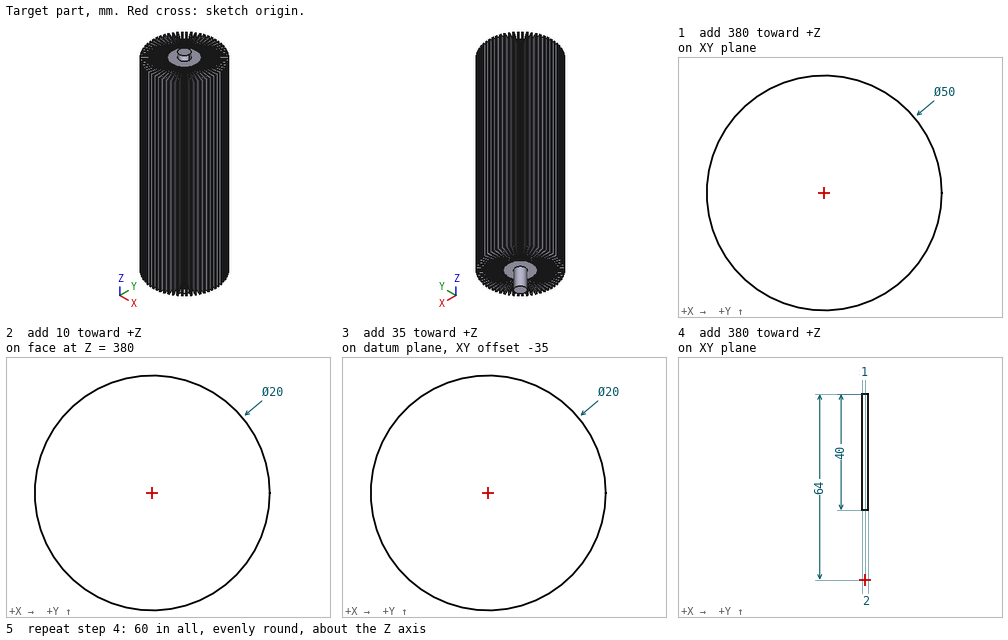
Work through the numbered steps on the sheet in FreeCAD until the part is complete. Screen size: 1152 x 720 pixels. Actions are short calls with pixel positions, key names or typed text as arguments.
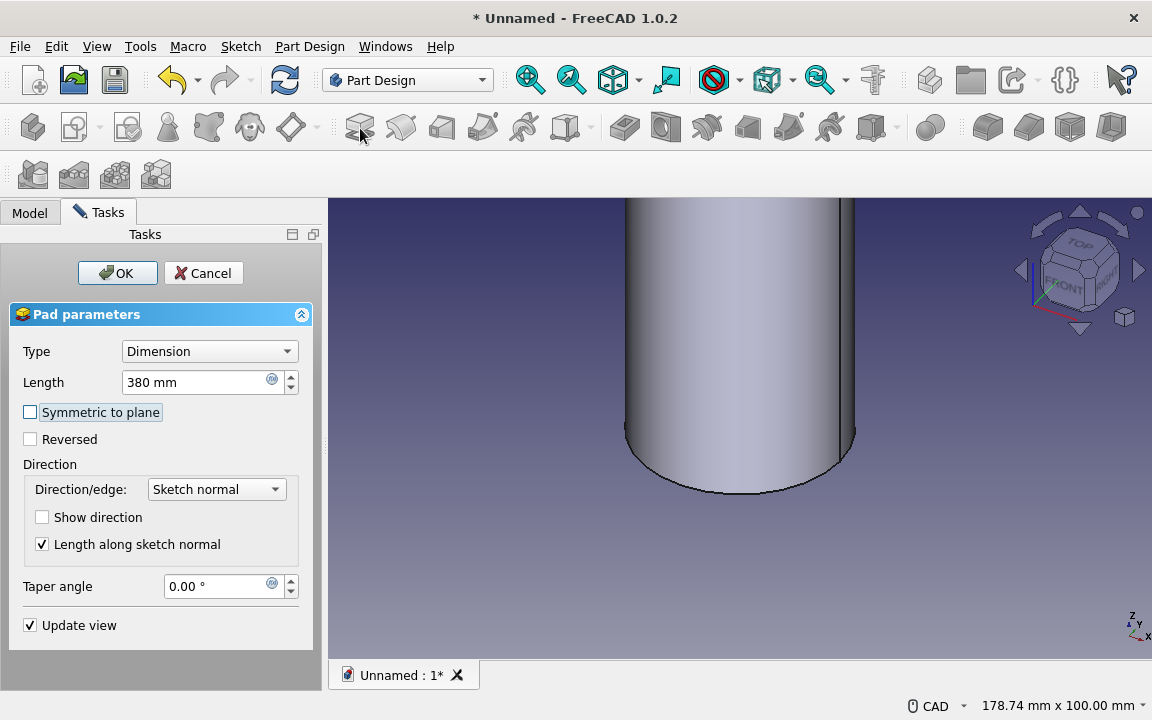
click(118, 273)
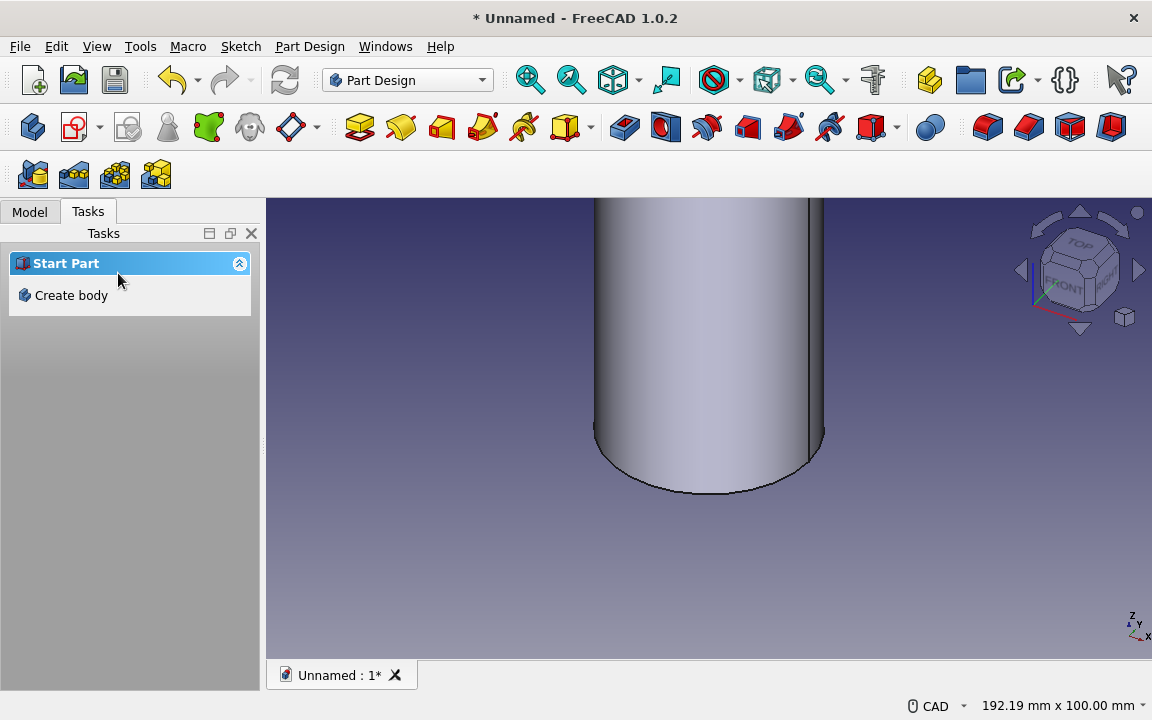
click(531, 80)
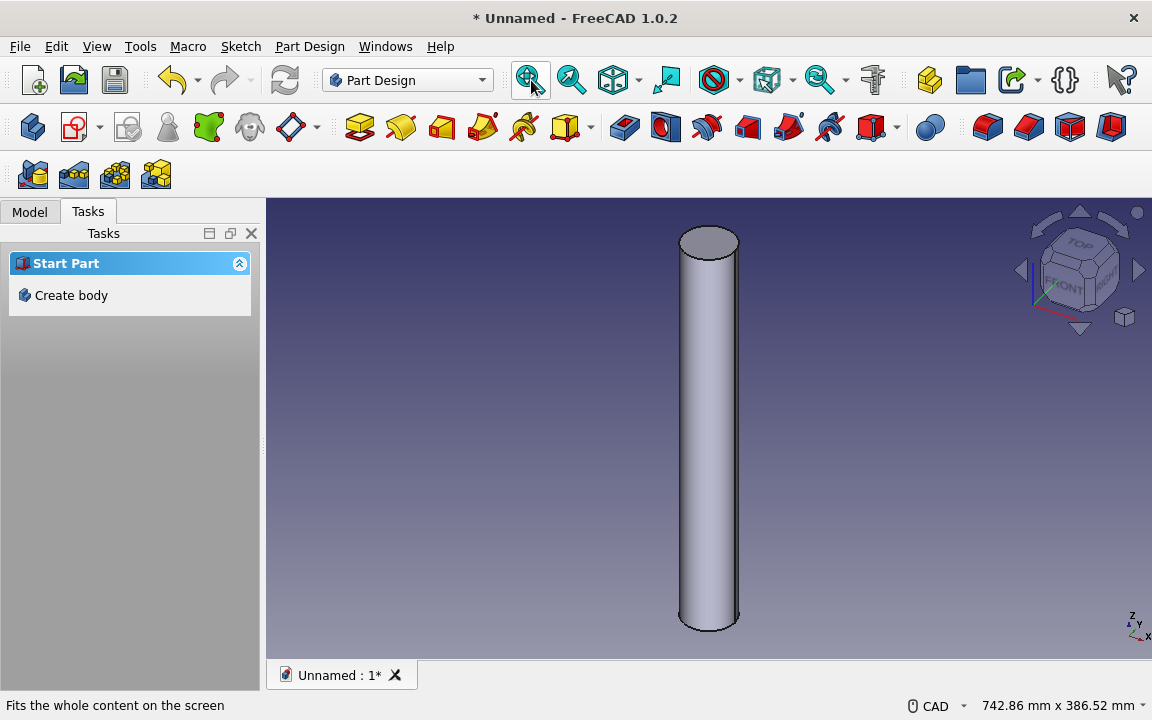
click(709, 242)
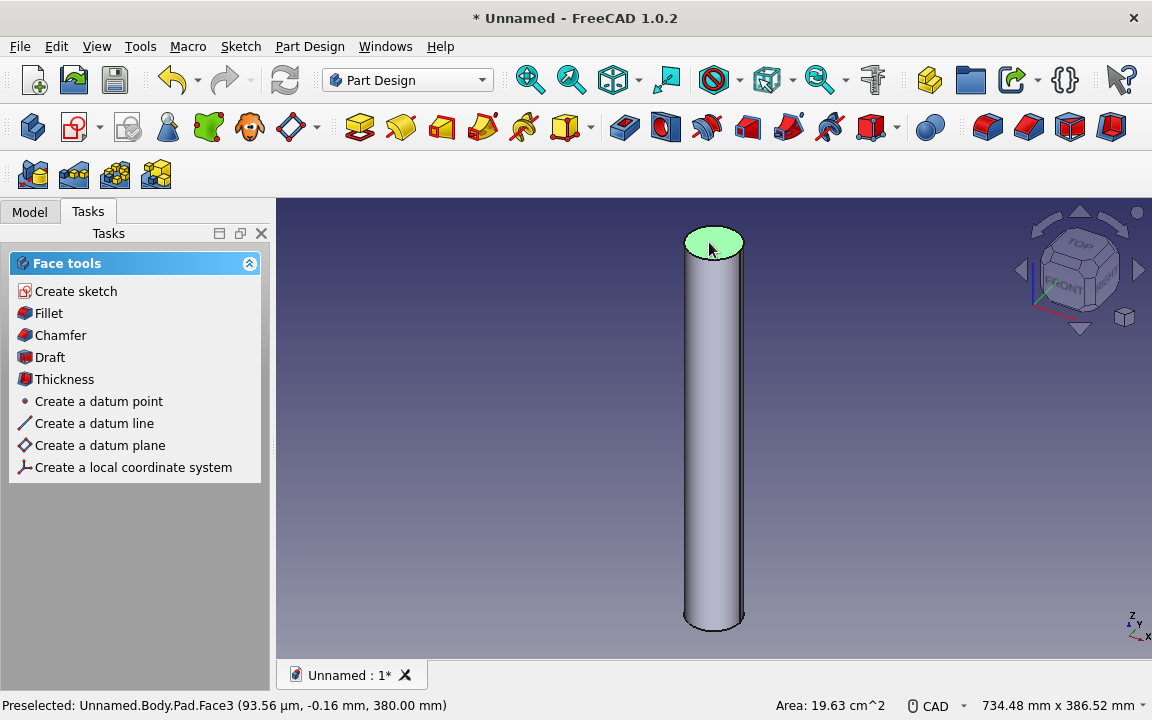
click(74, 128)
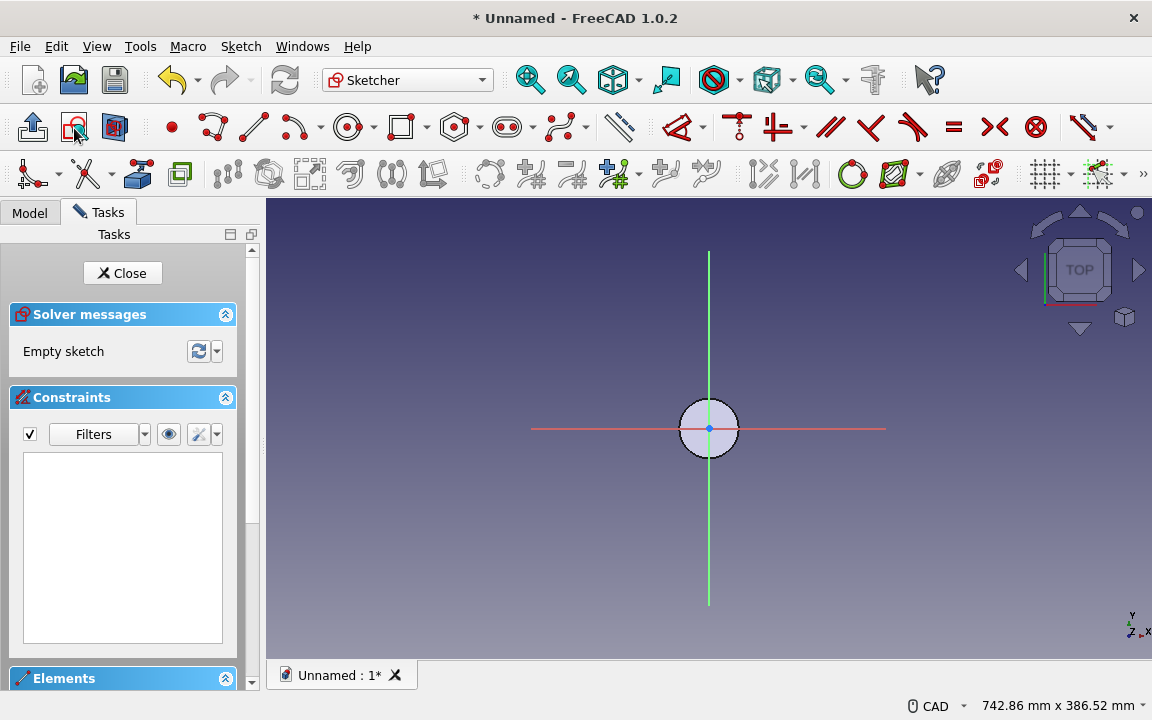
scroll(716, 428, up, 12)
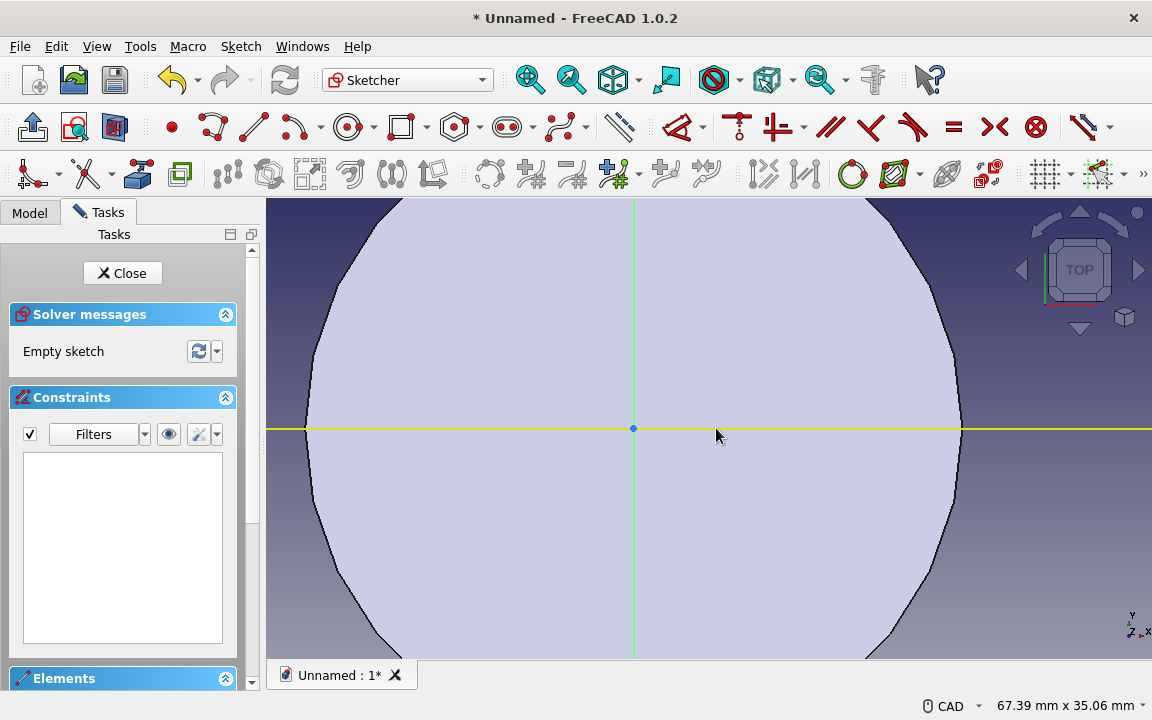
click(348, 128)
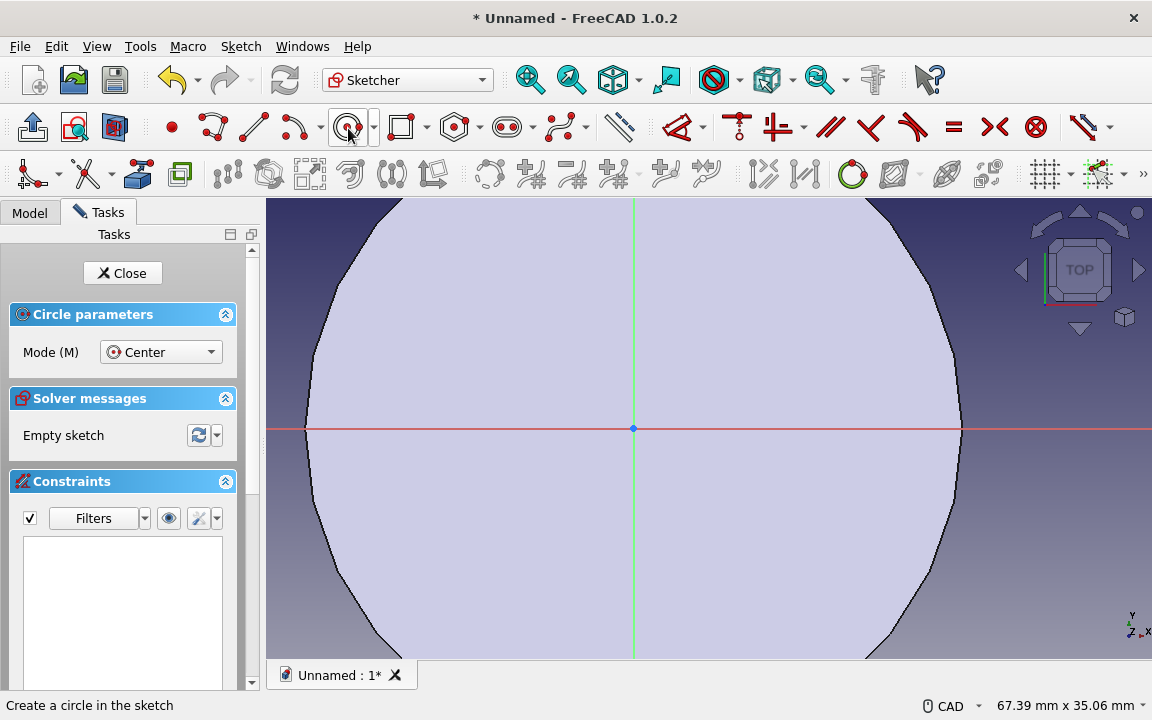
click(634, 428)
click(727, 336)
key(Escape)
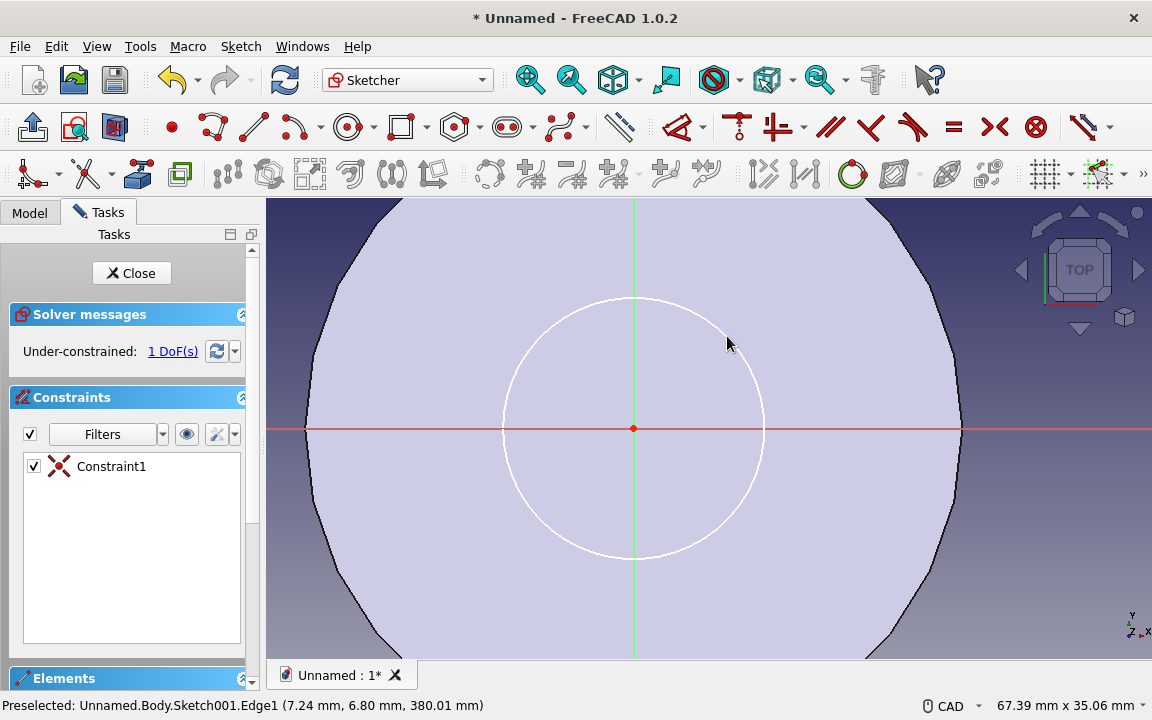
key(d)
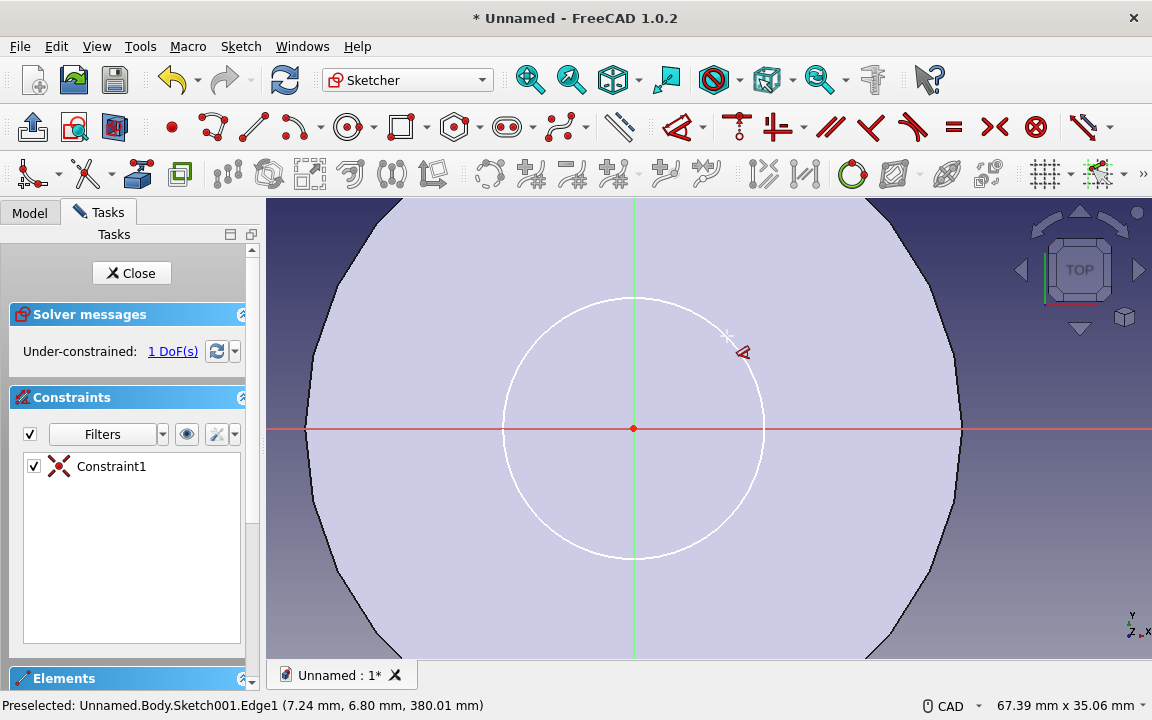
click(726, 336)
click(749, 313)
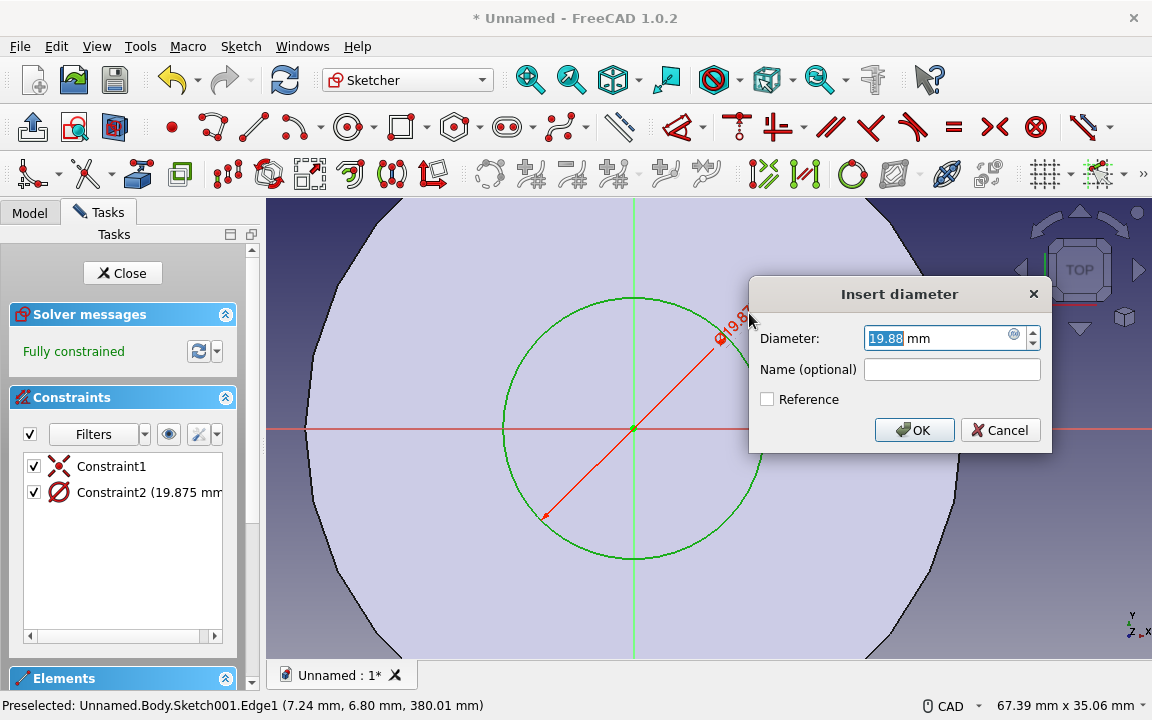
text(20)
key(Return)
key(Escape)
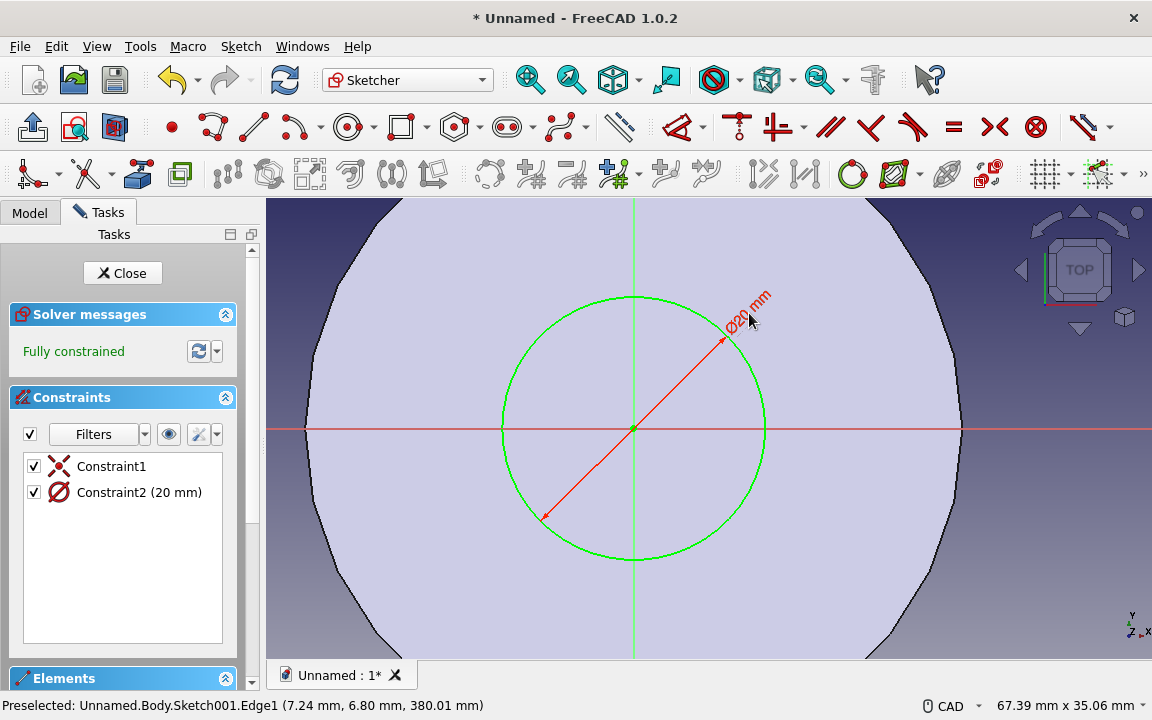
click(123, 273)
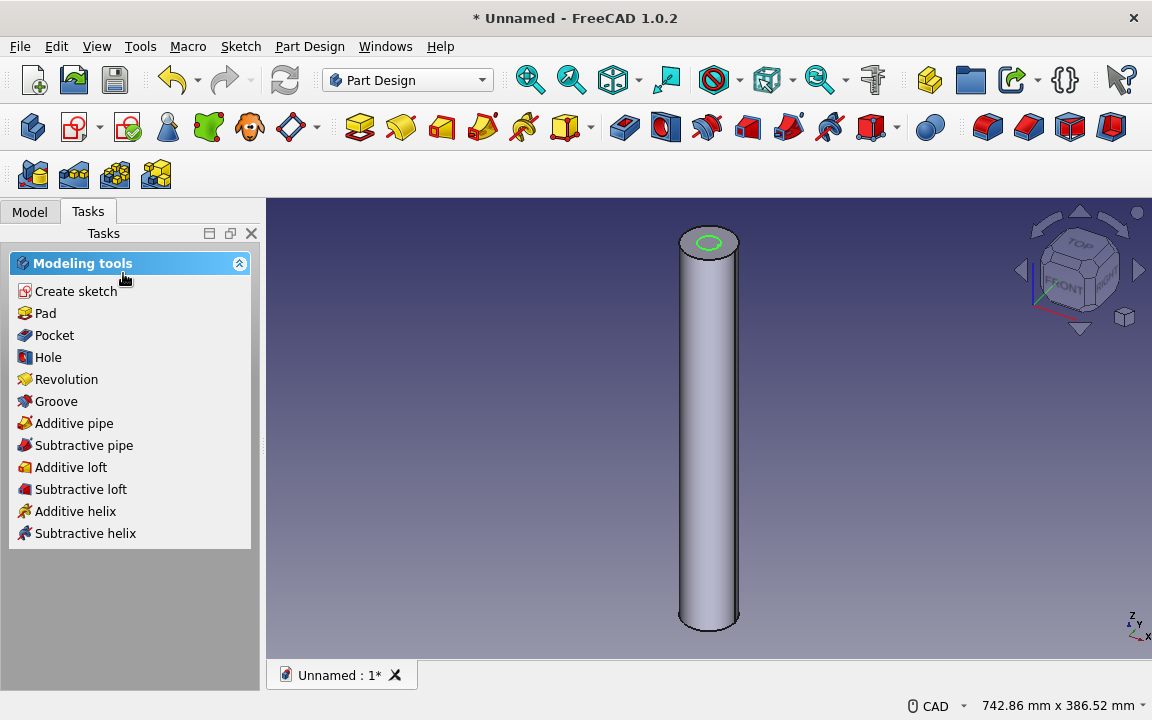
click(360, 128)